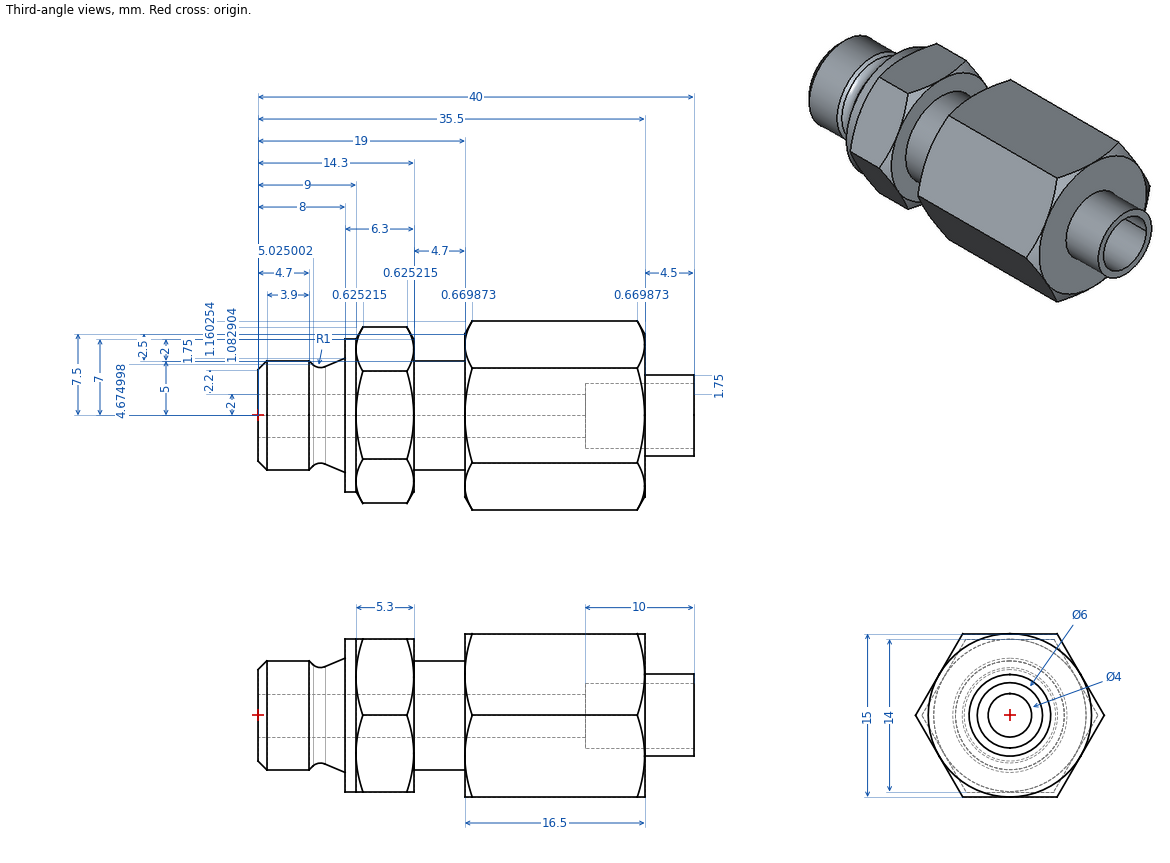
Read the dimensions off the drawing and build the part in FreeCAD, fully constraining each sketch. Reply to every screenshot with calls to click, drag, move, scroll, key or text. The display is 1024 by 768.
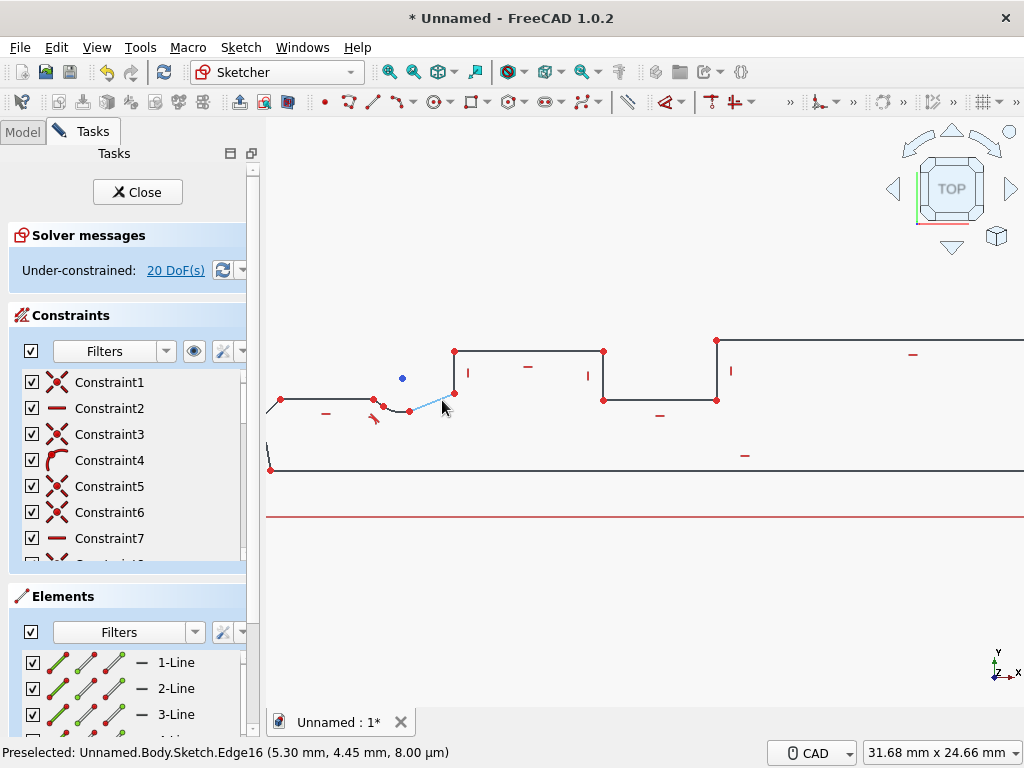
click(441, 399)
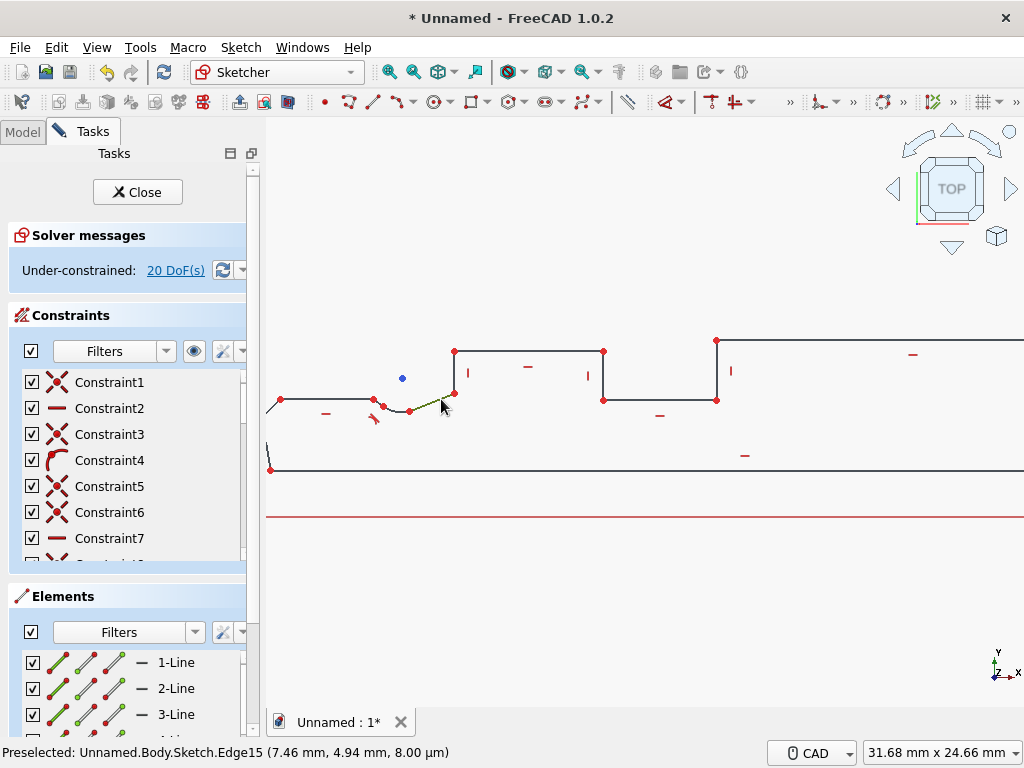
click(395, 412)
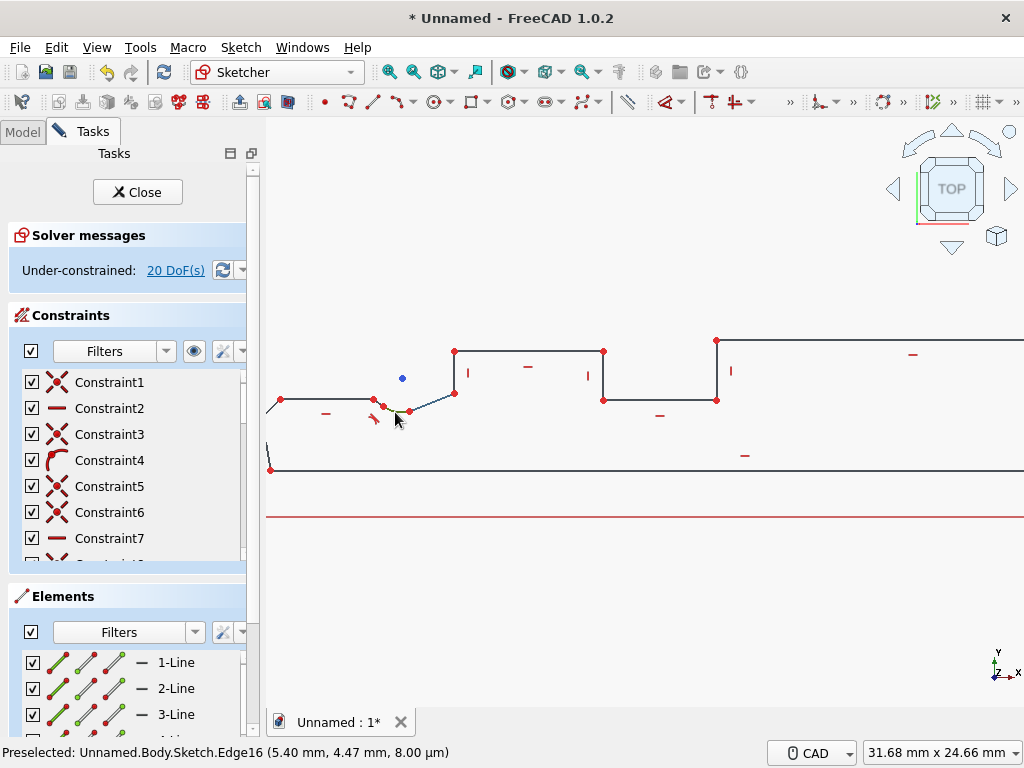
key(t)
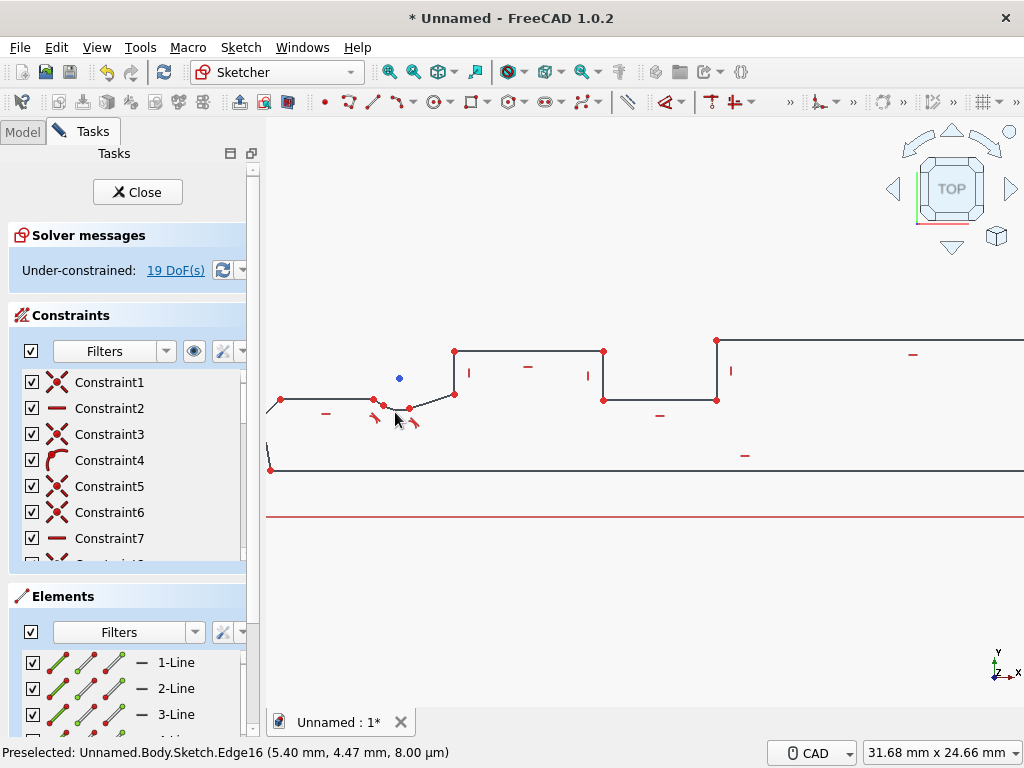
scroll(443, 399, down, 4)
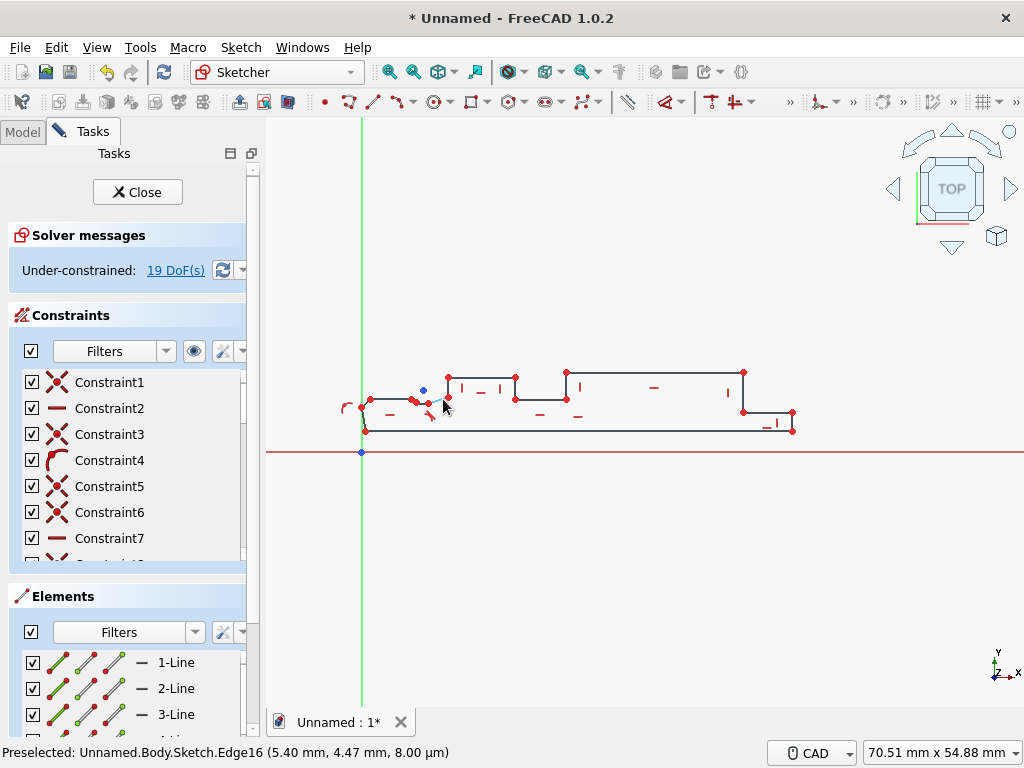
scroll(363, 415, up, 4)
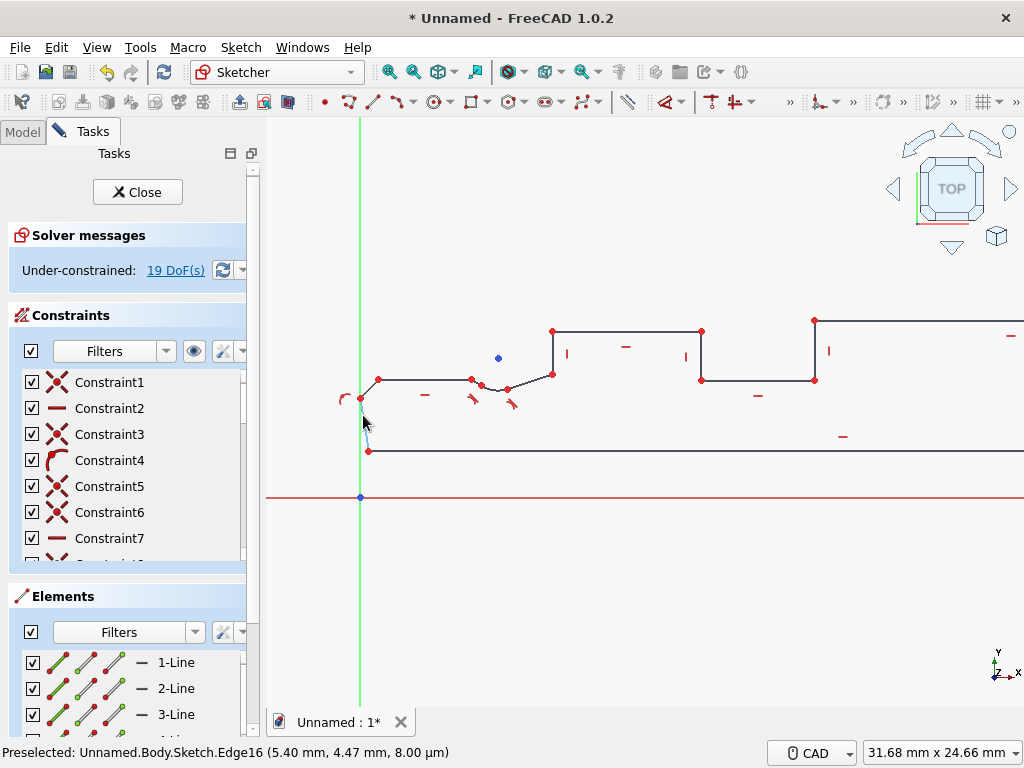
click(363, 414)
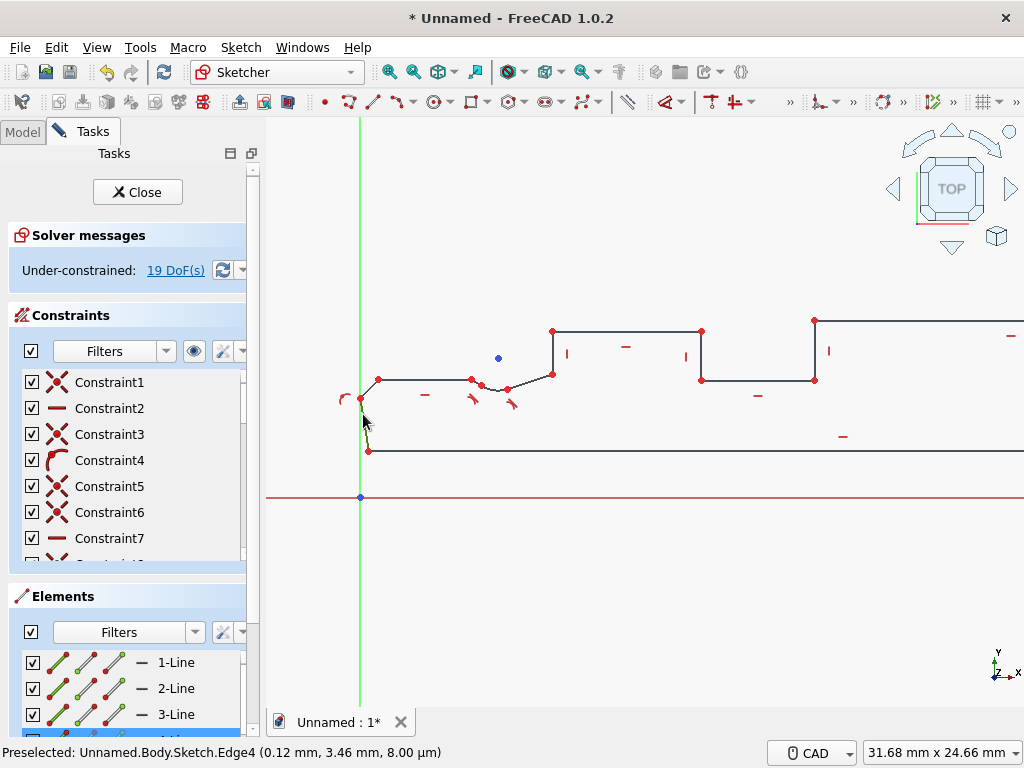
key(v)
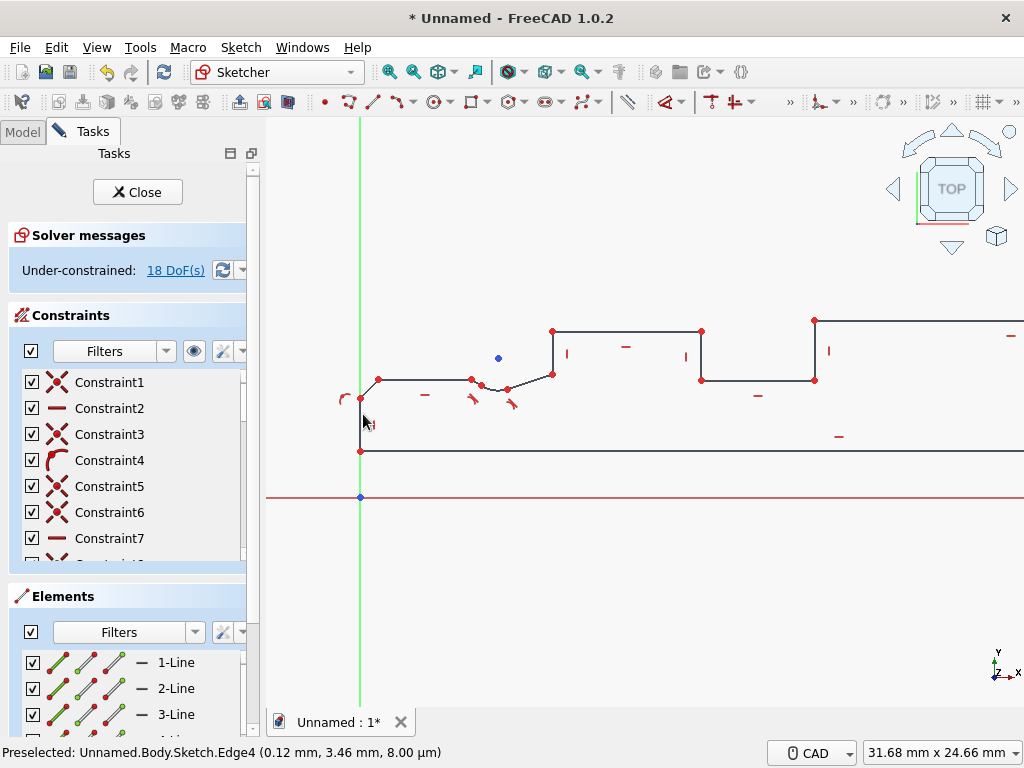
key(d)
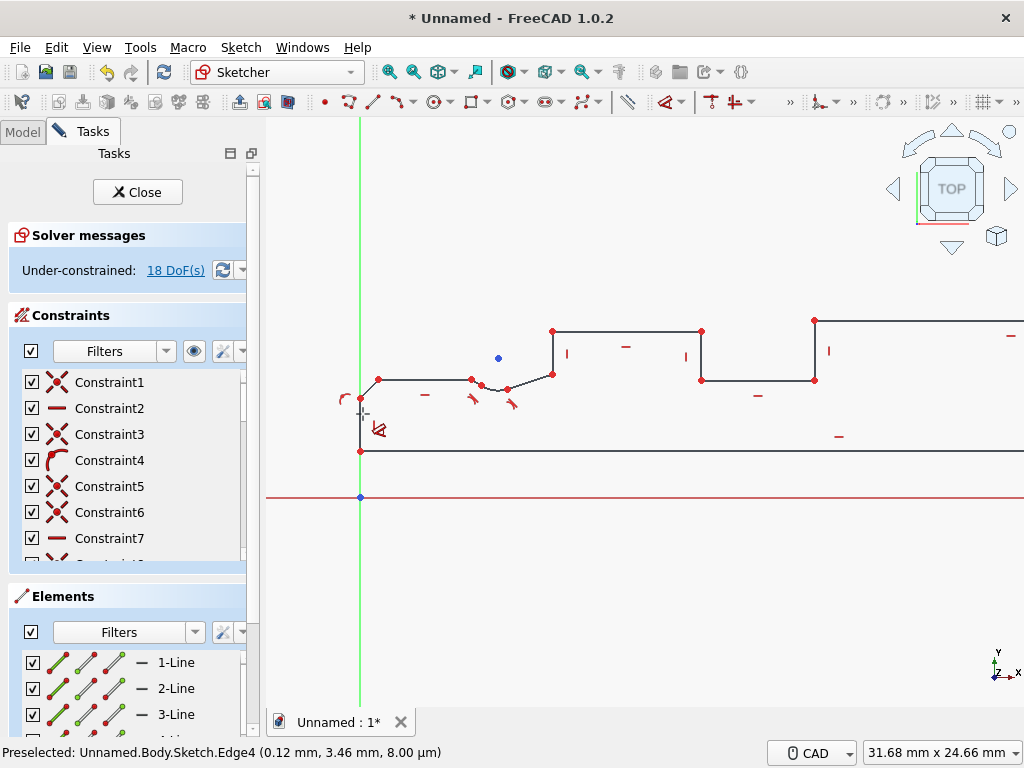
scroll(494, 390, up, 3)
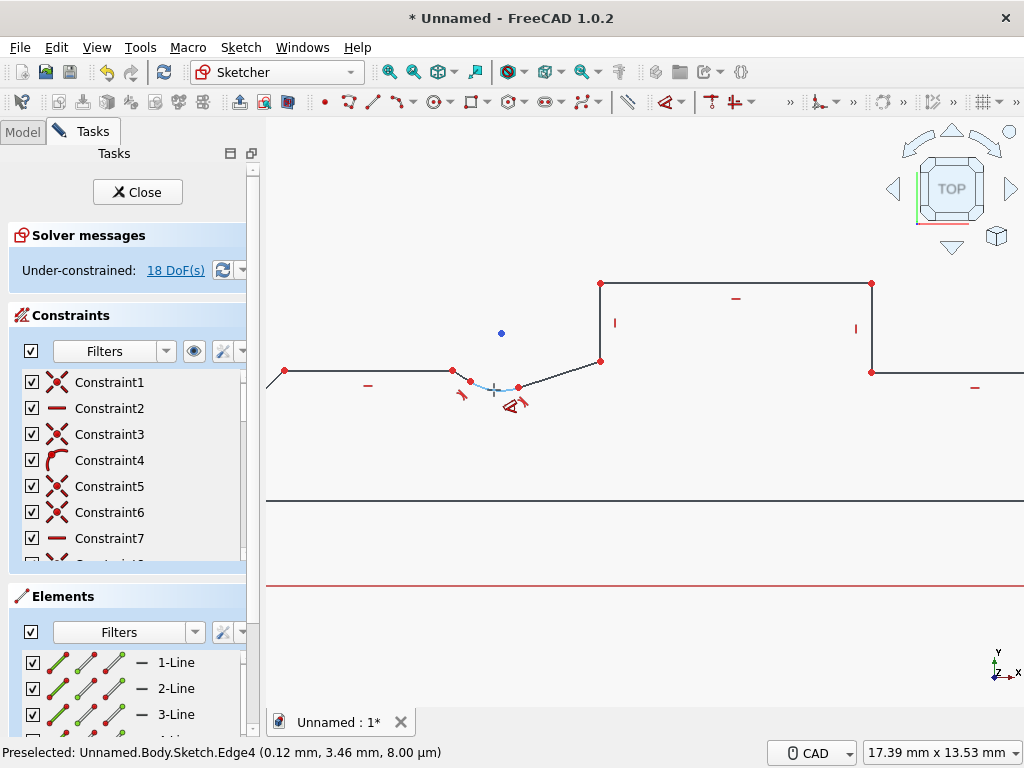
click(494, 390)
click(490, 422)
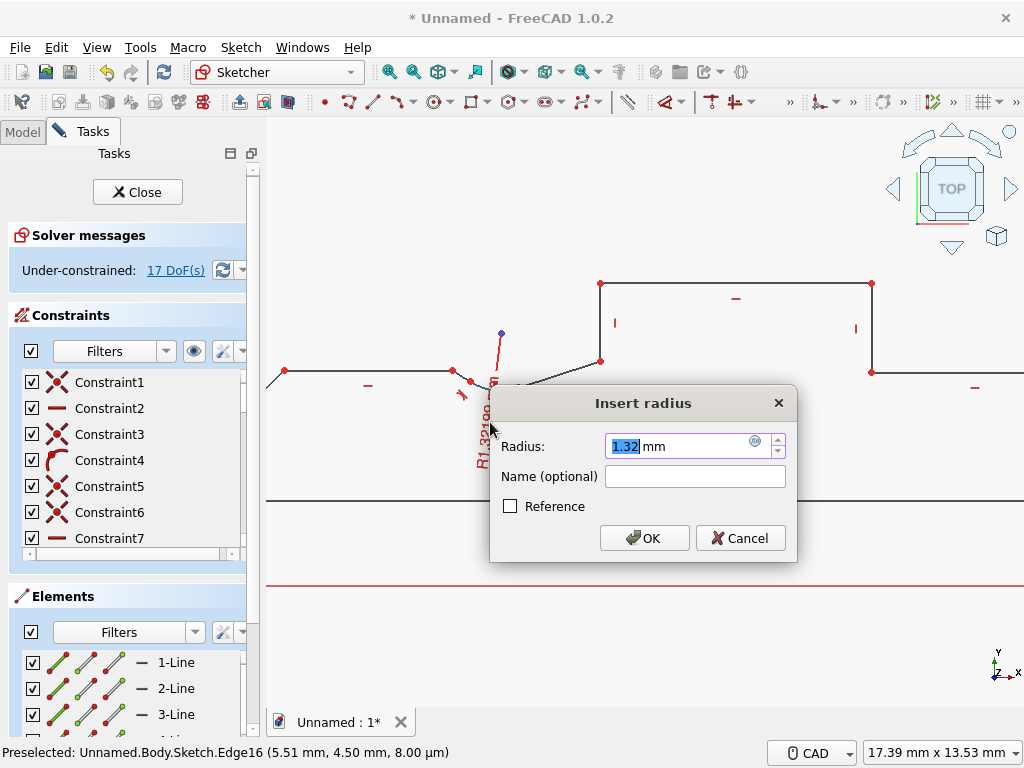
text(1)
key(Return)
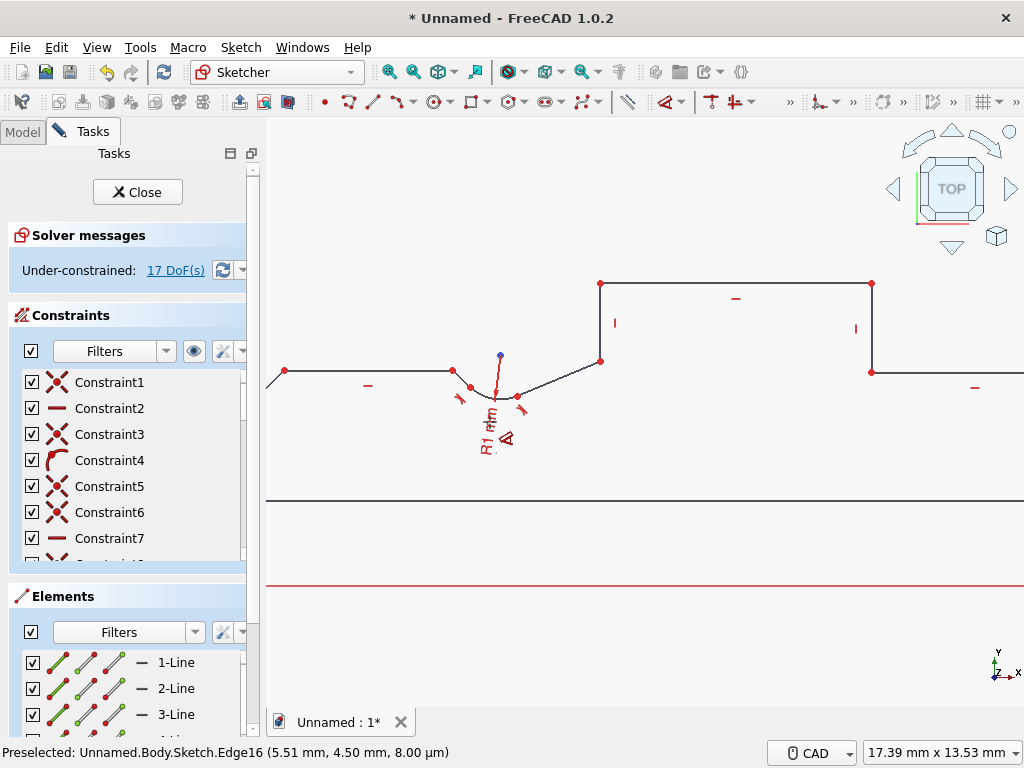
scroll(398, 409, down, 7)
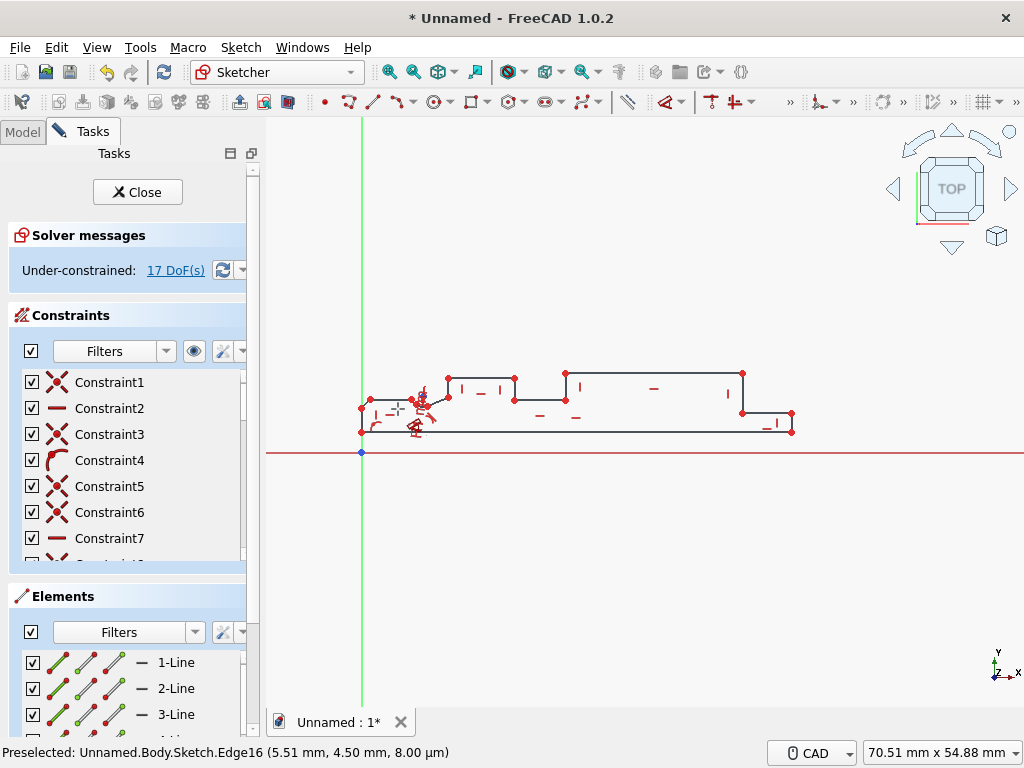
scroll(515, 394, up, 4)